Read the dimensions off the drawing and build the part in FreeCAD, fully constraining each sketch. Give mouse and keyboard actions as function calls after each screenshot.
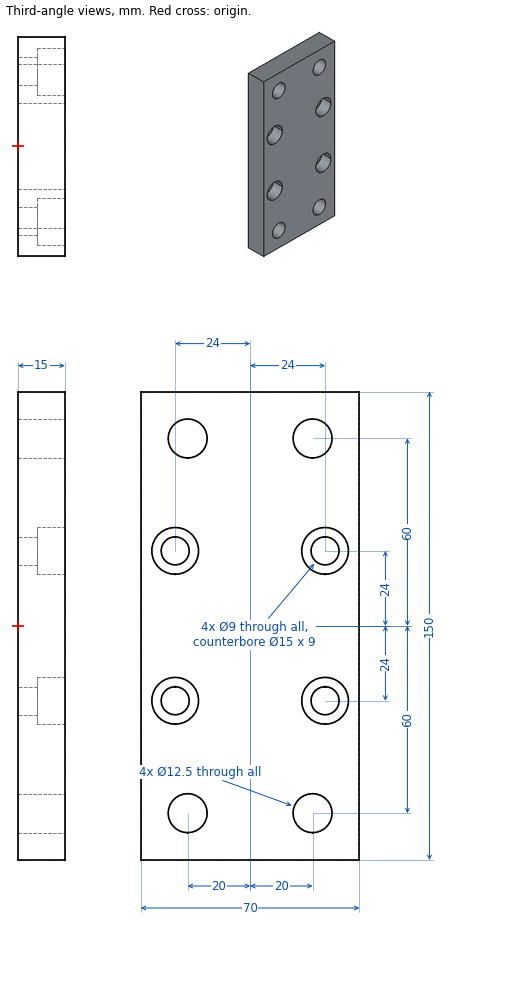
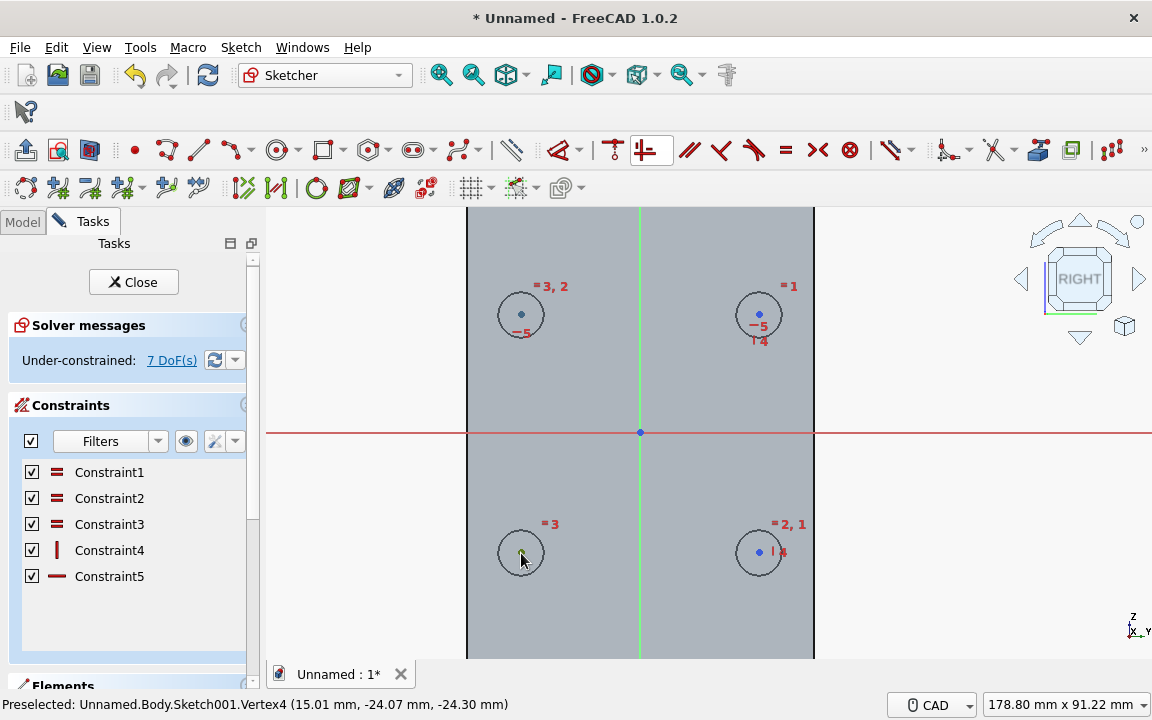
key(v)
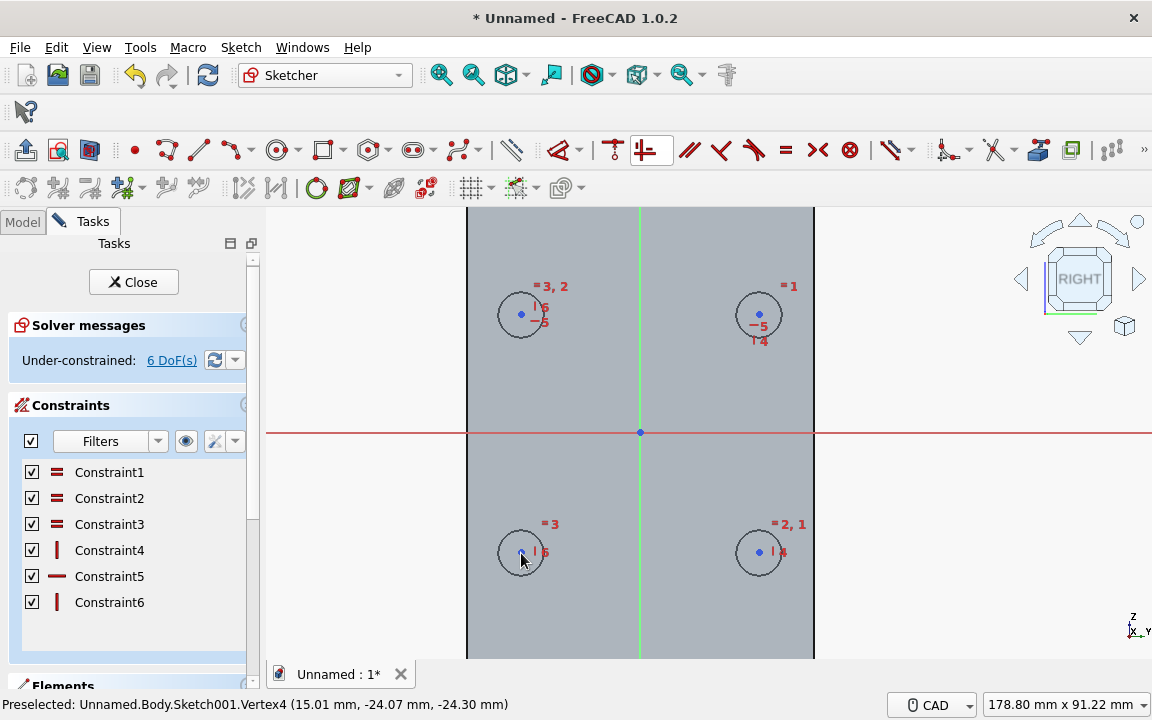
click(759, 553)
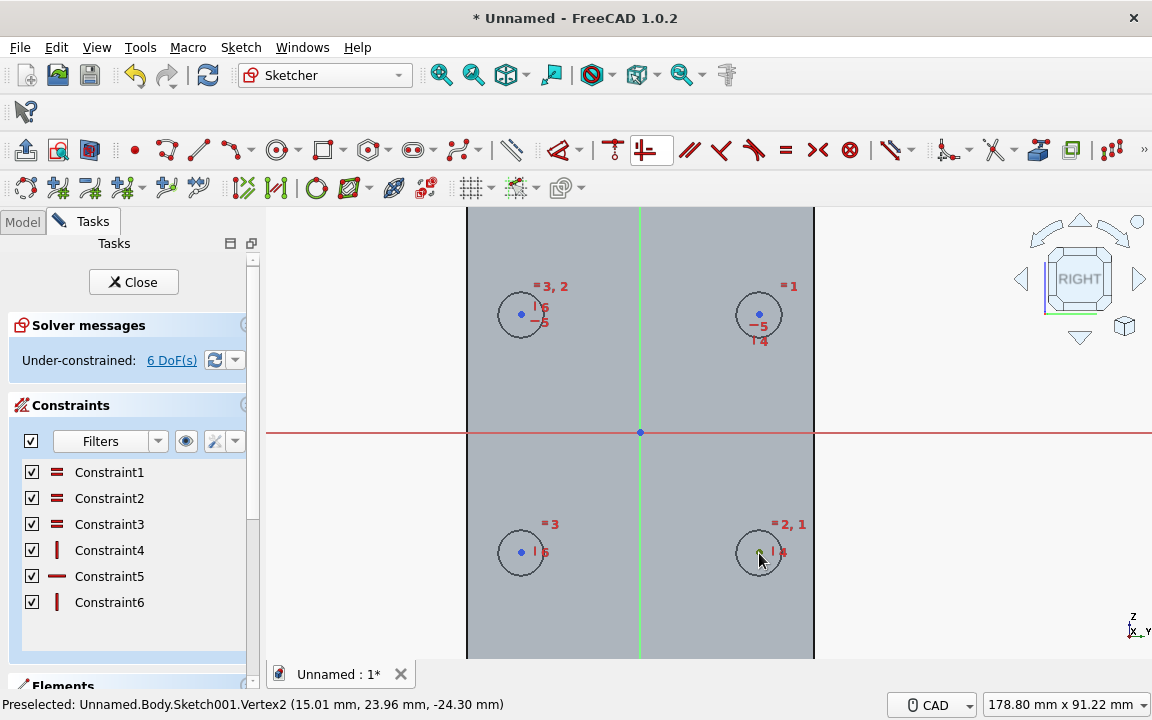
click(521, 553)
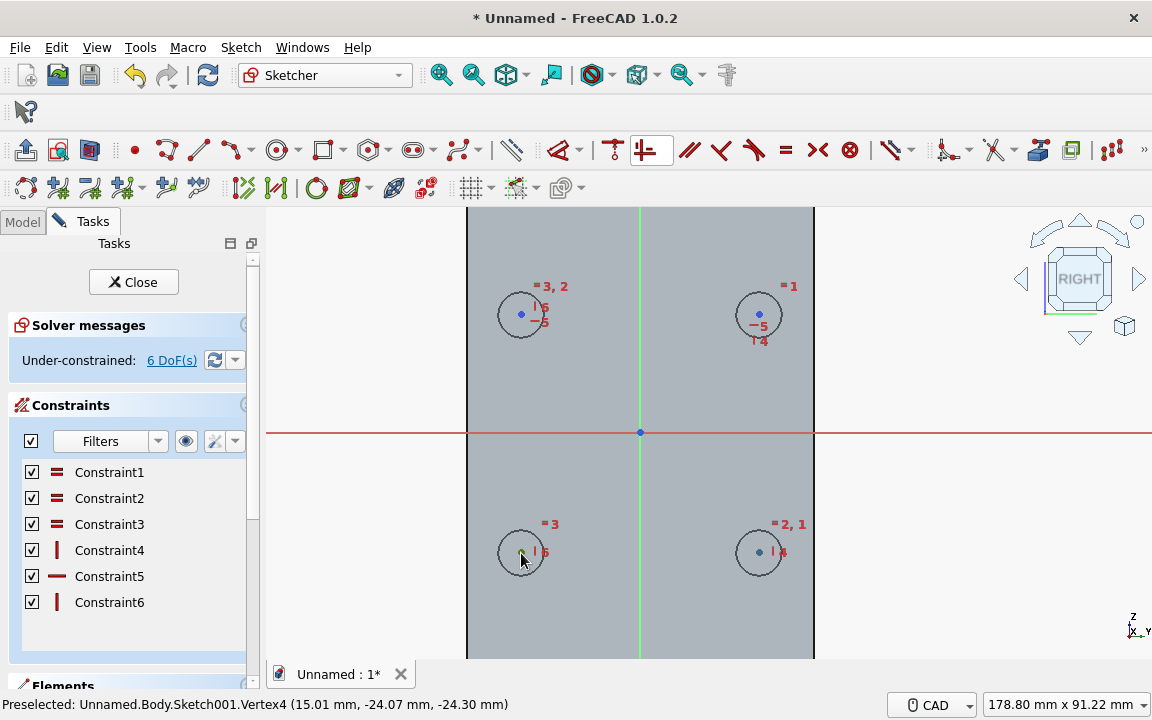
key(h)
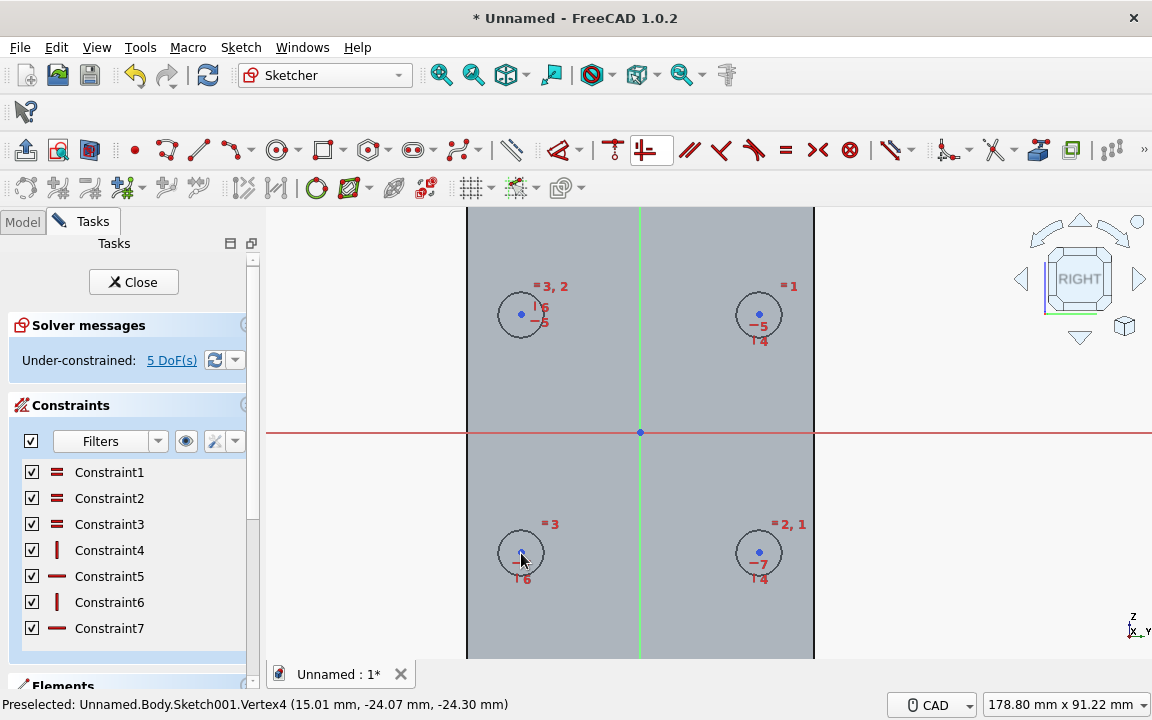
key(d)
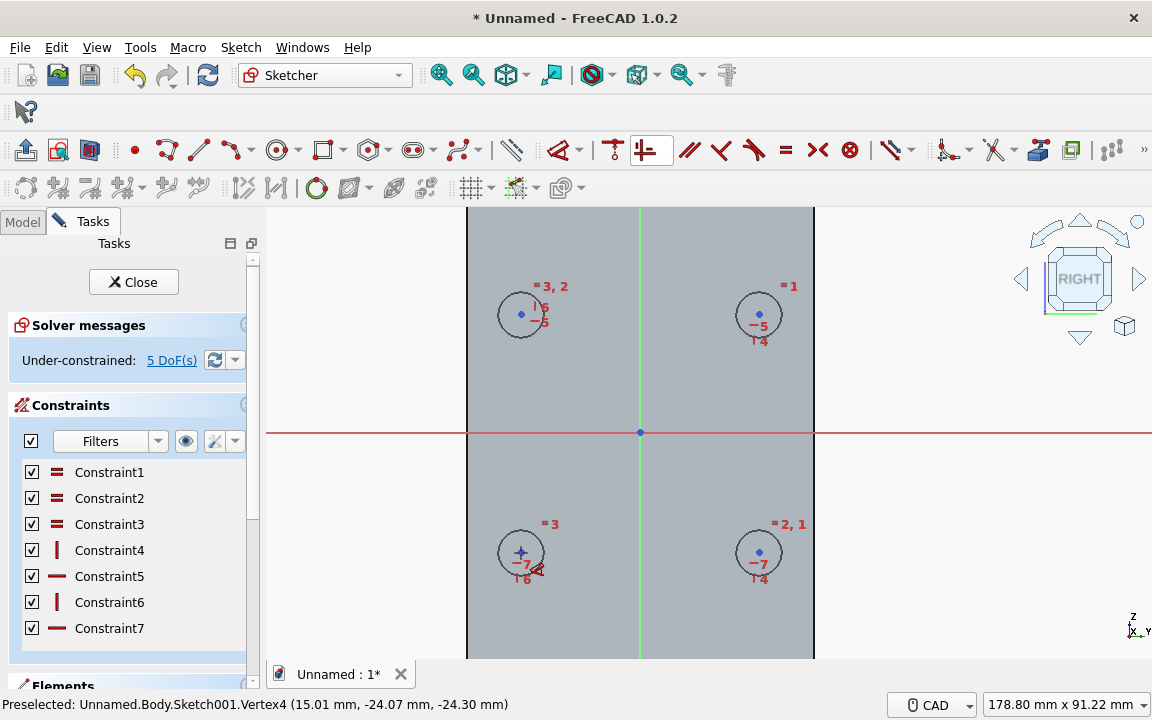
click(775, 299)
click(798, 276)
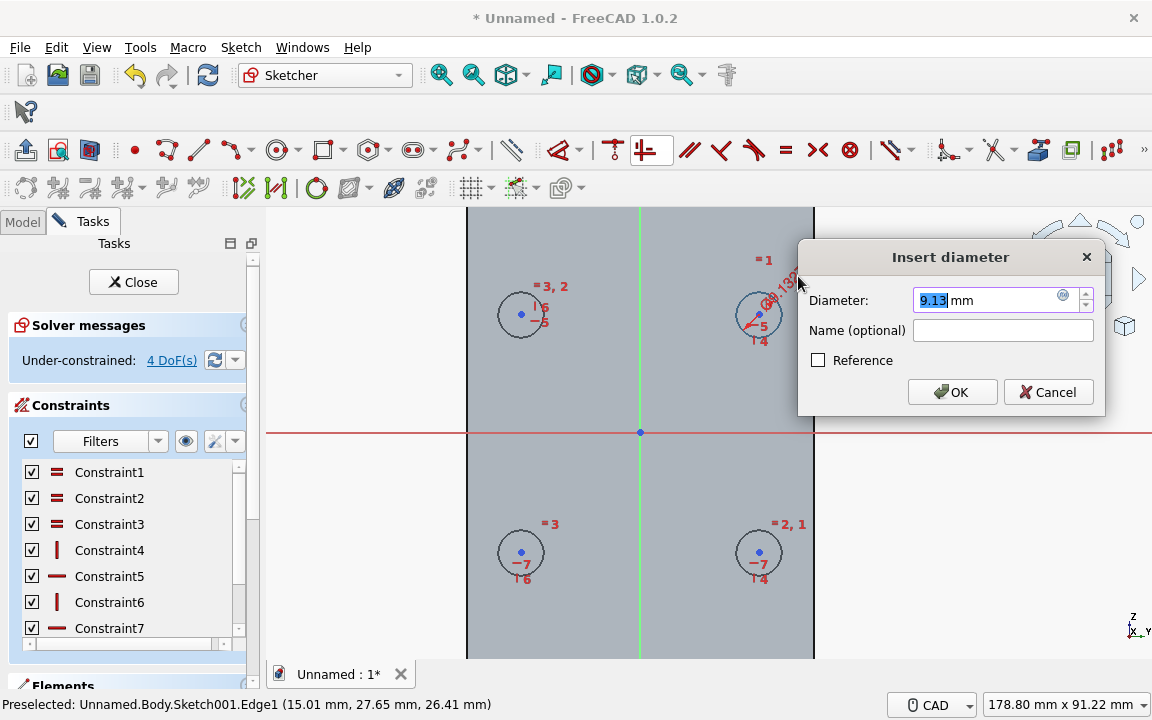
text(9)
key(Return)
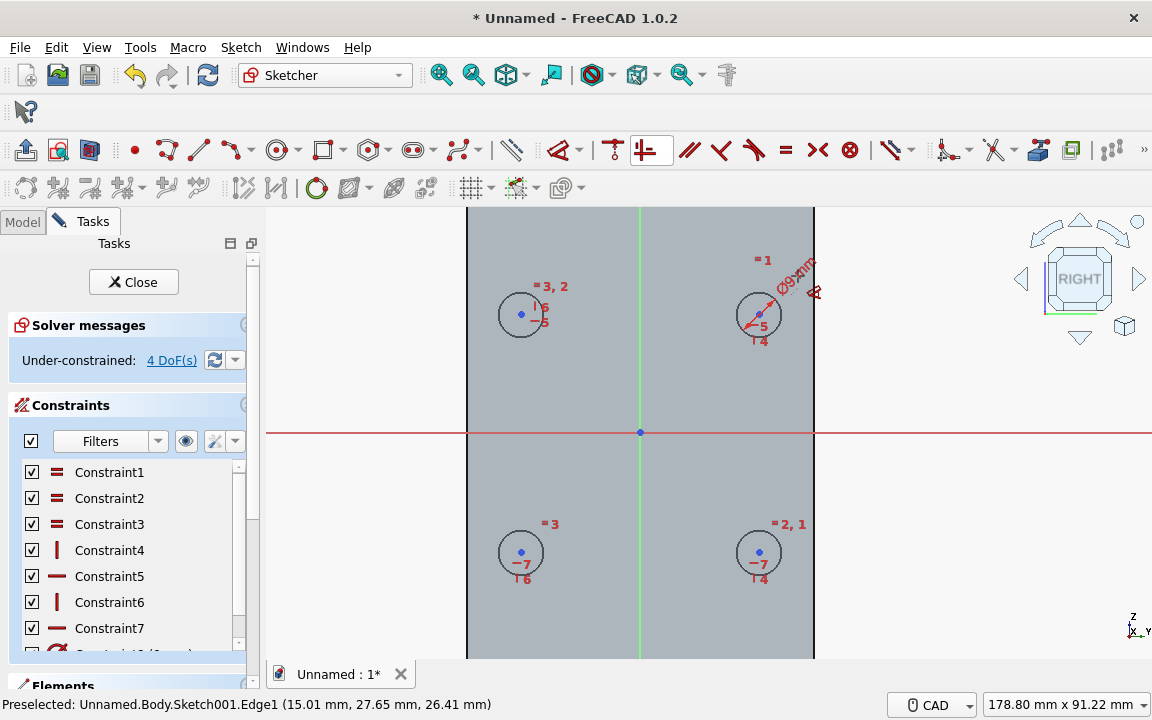
click(759, 315)
click(700, 281)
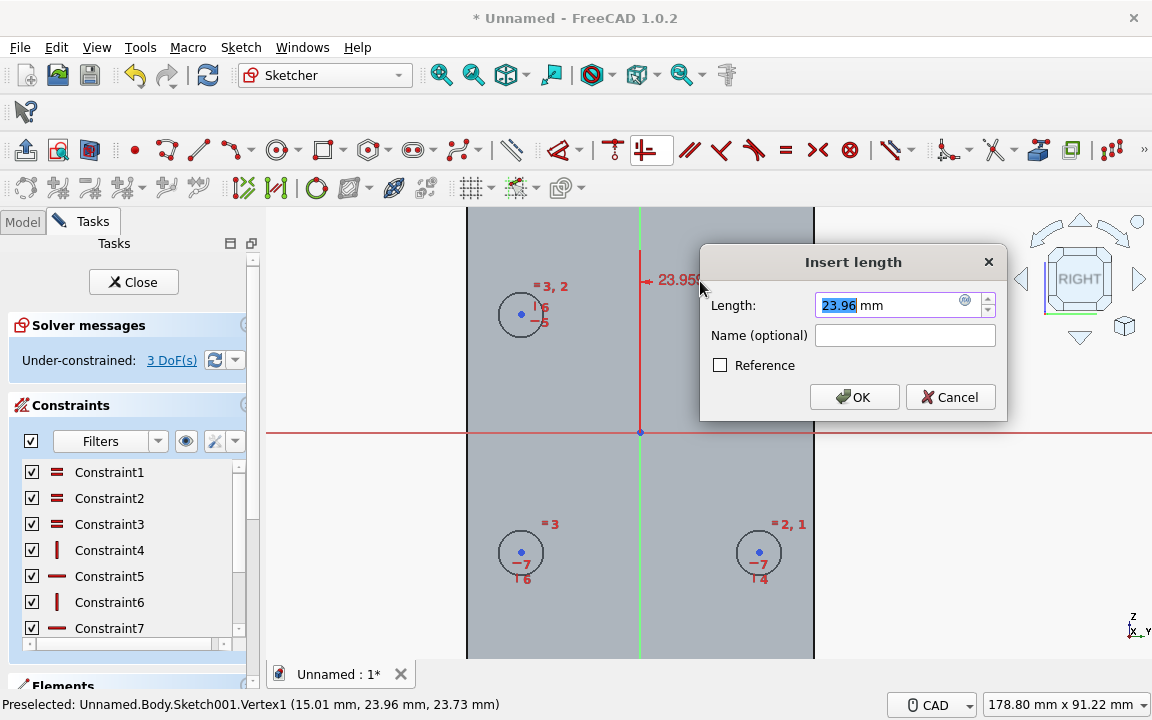
text(24)
key(Return)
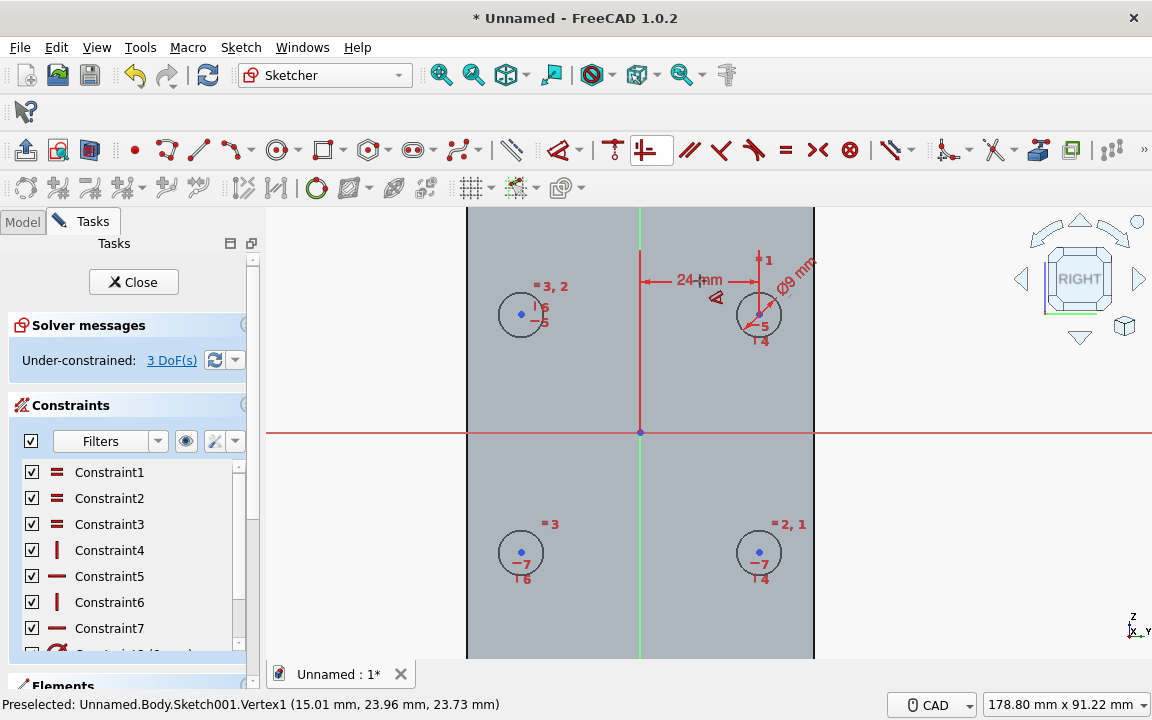
click(759, 315)
click(793, 374)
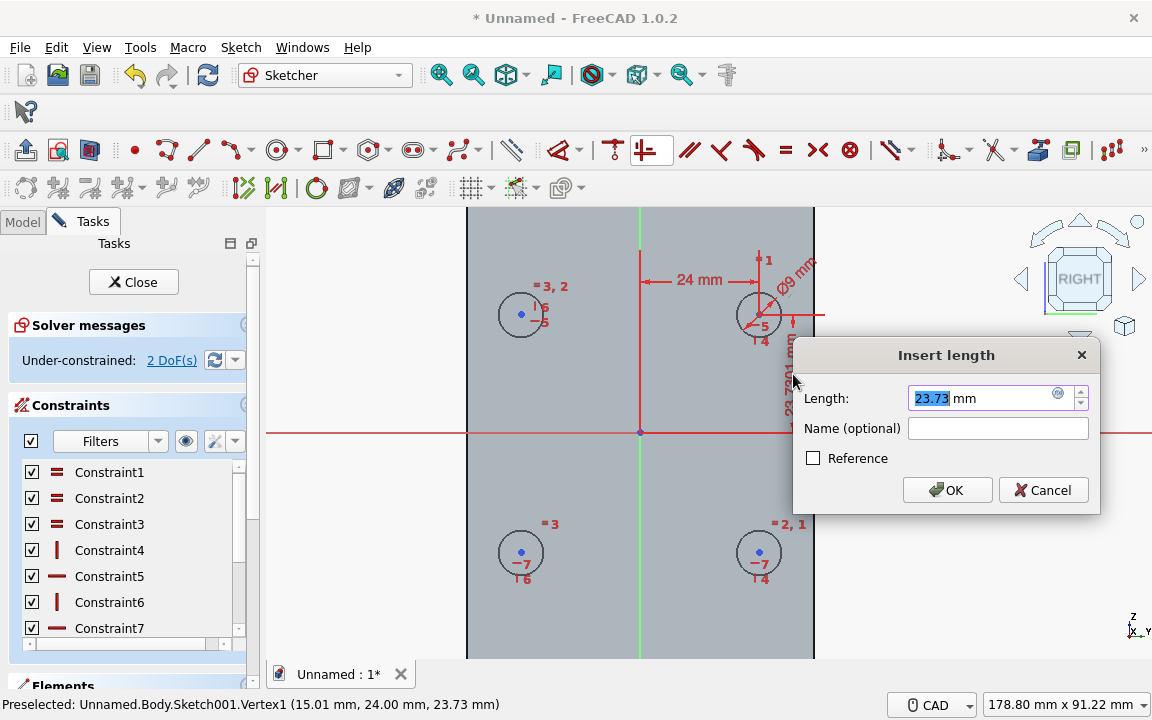
text(24)
key(Return)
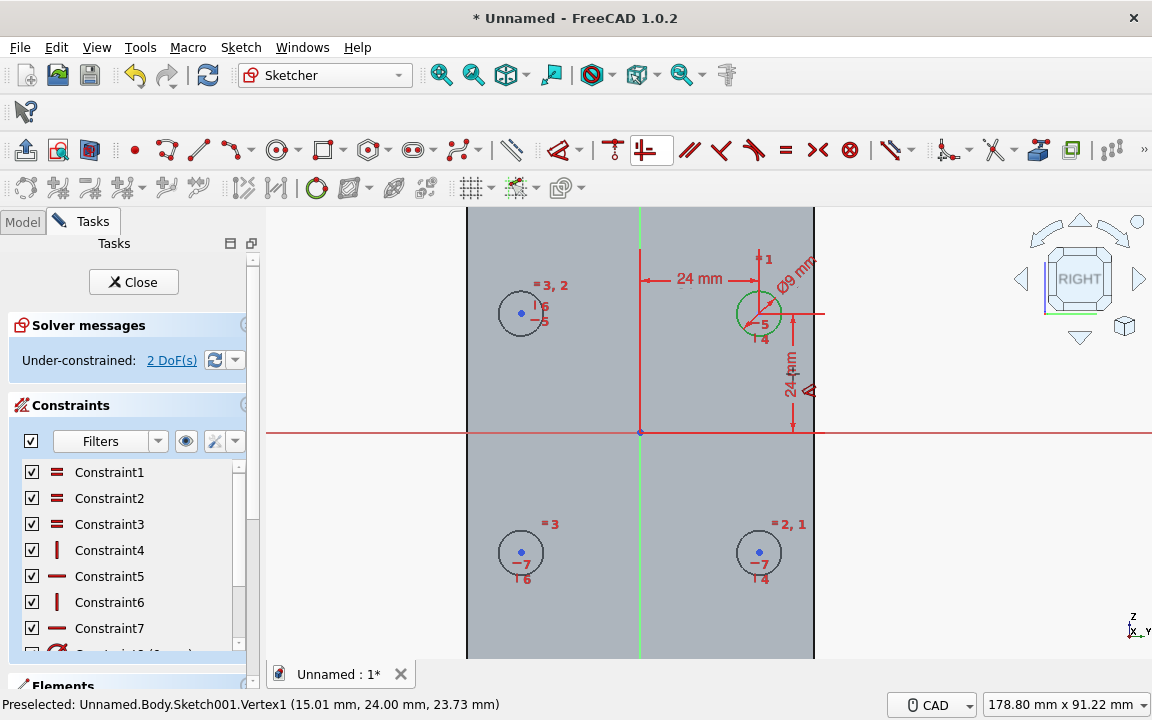
click(759, 553)
click(793, 493)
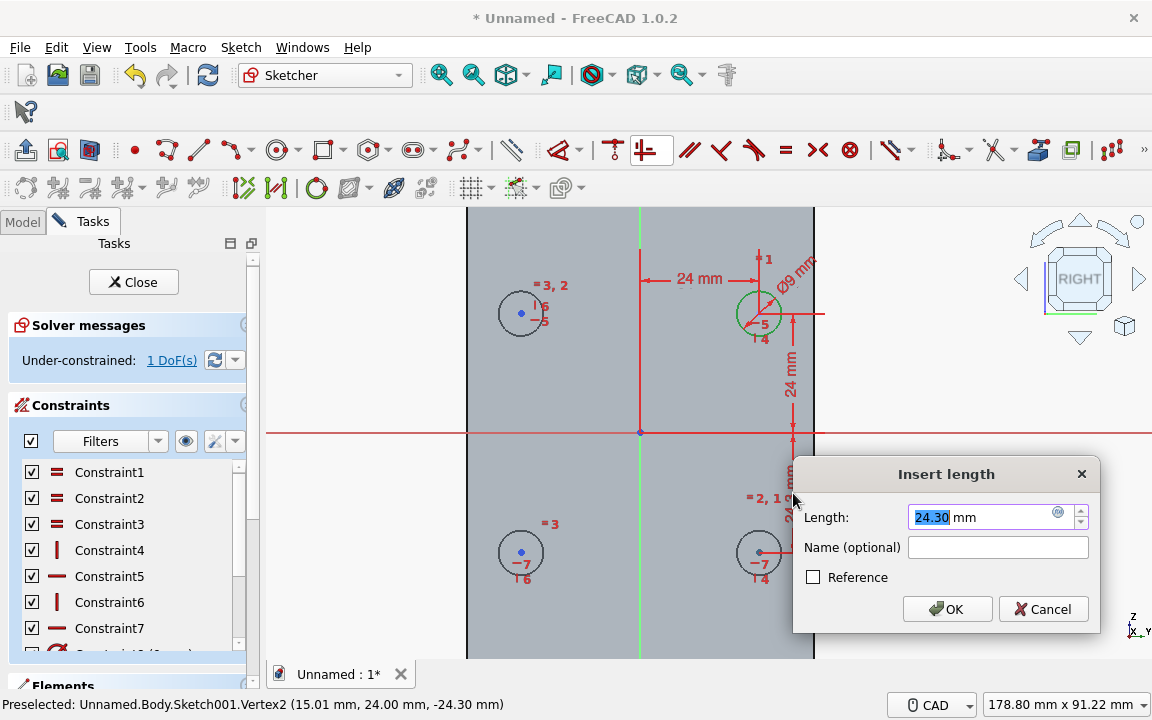
text(24)
key(Return)